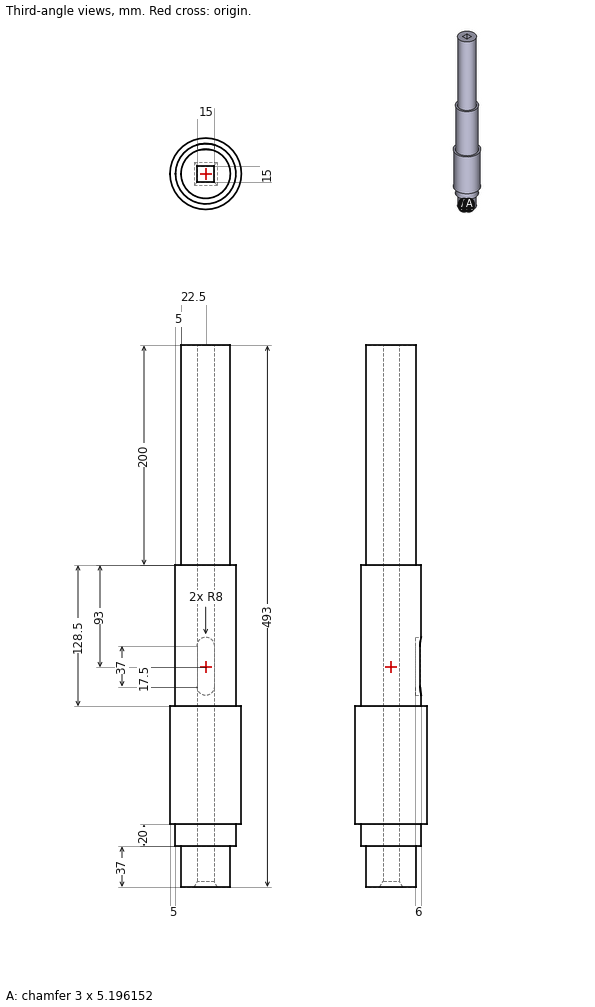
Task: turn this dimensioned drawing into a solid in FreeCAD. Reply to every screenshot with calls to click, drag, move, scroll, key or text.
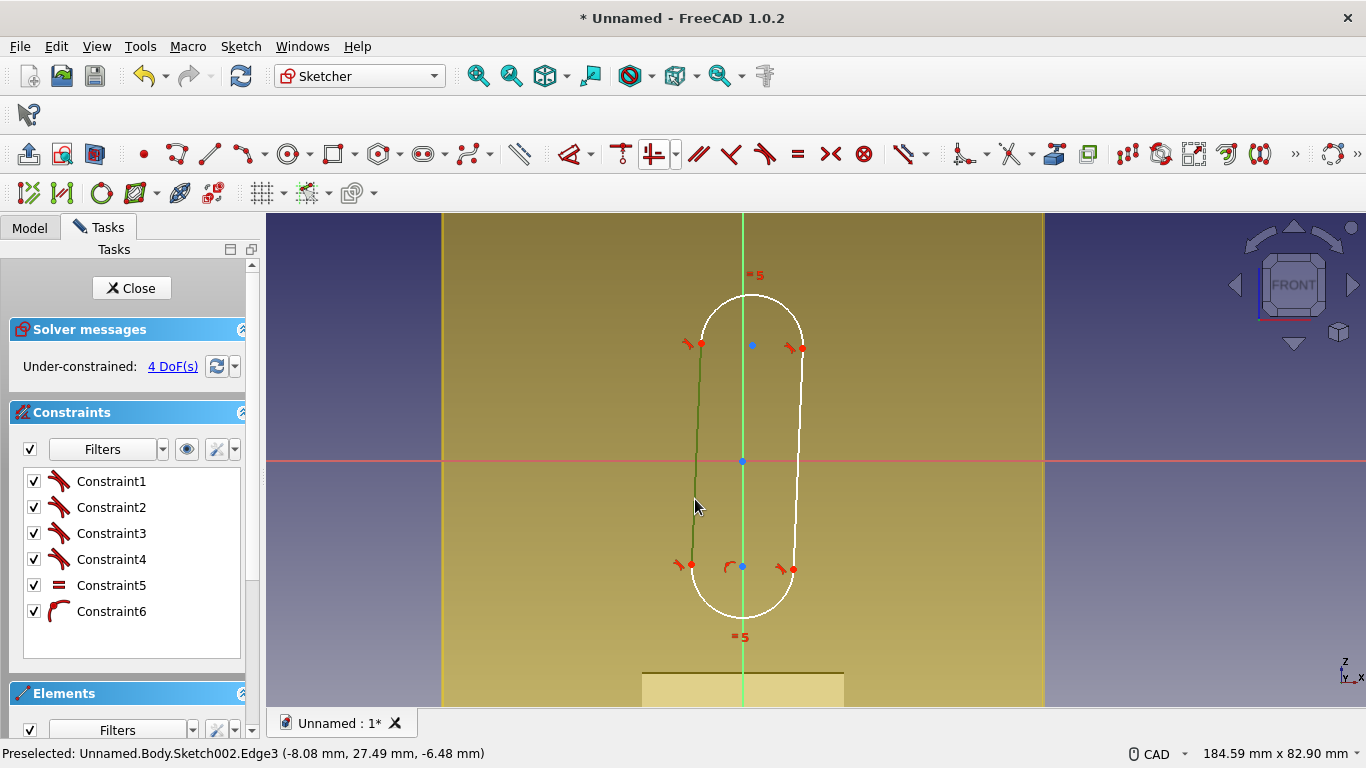
key(v)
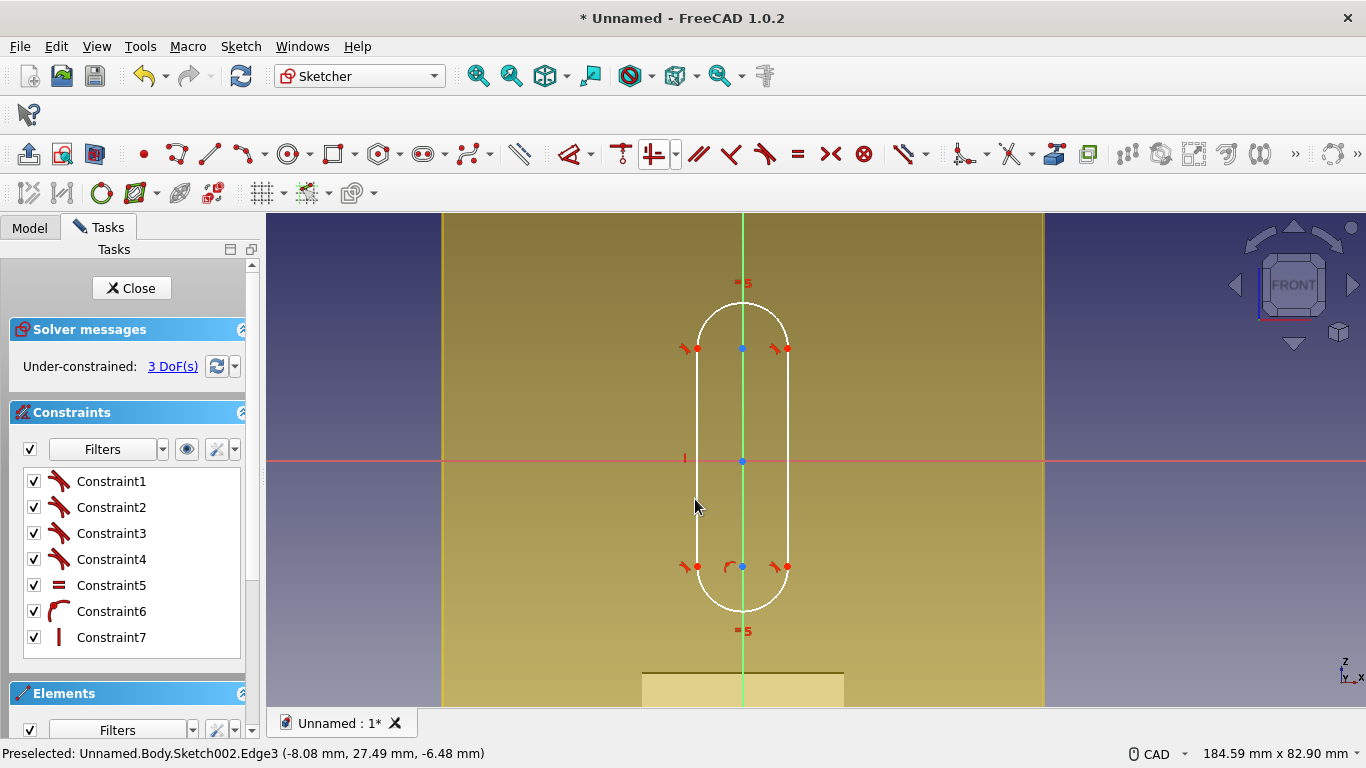
key(d)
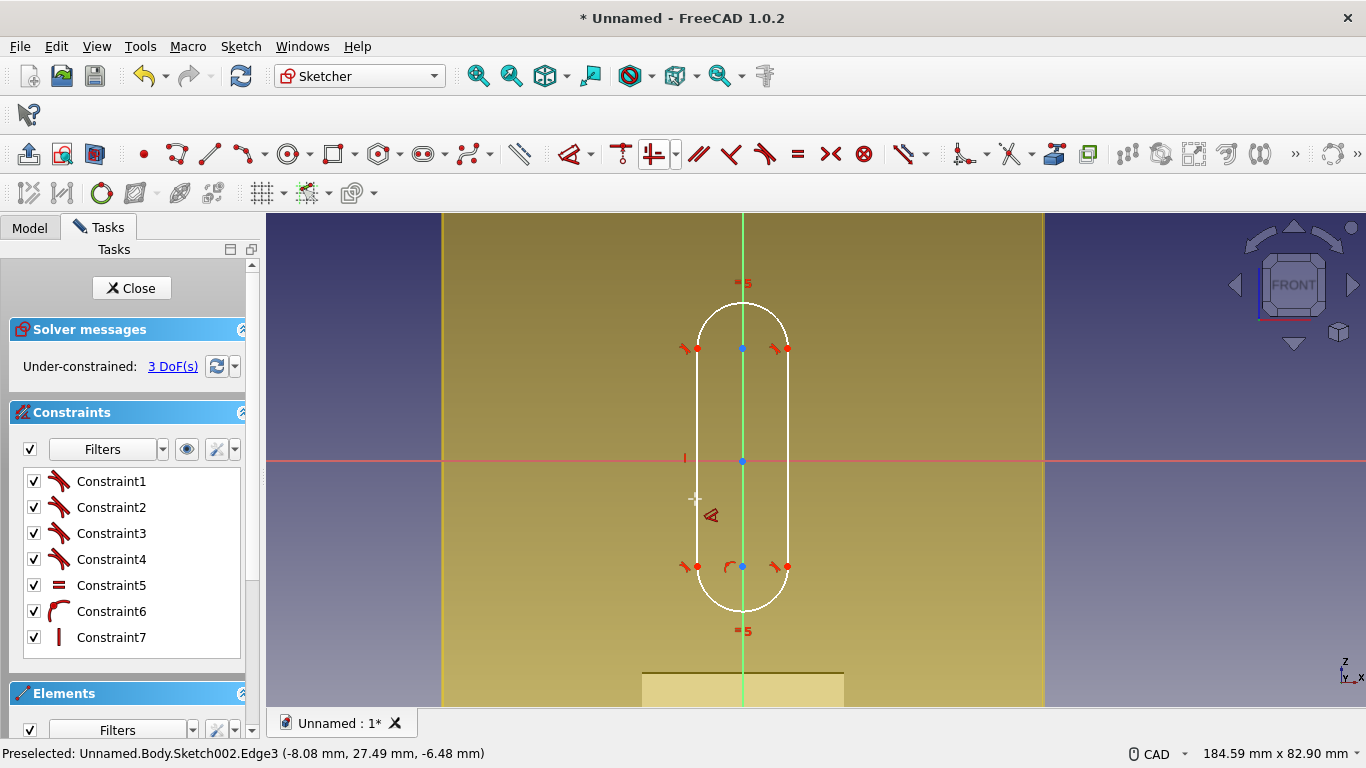
click(716, 603)
click(697, 629)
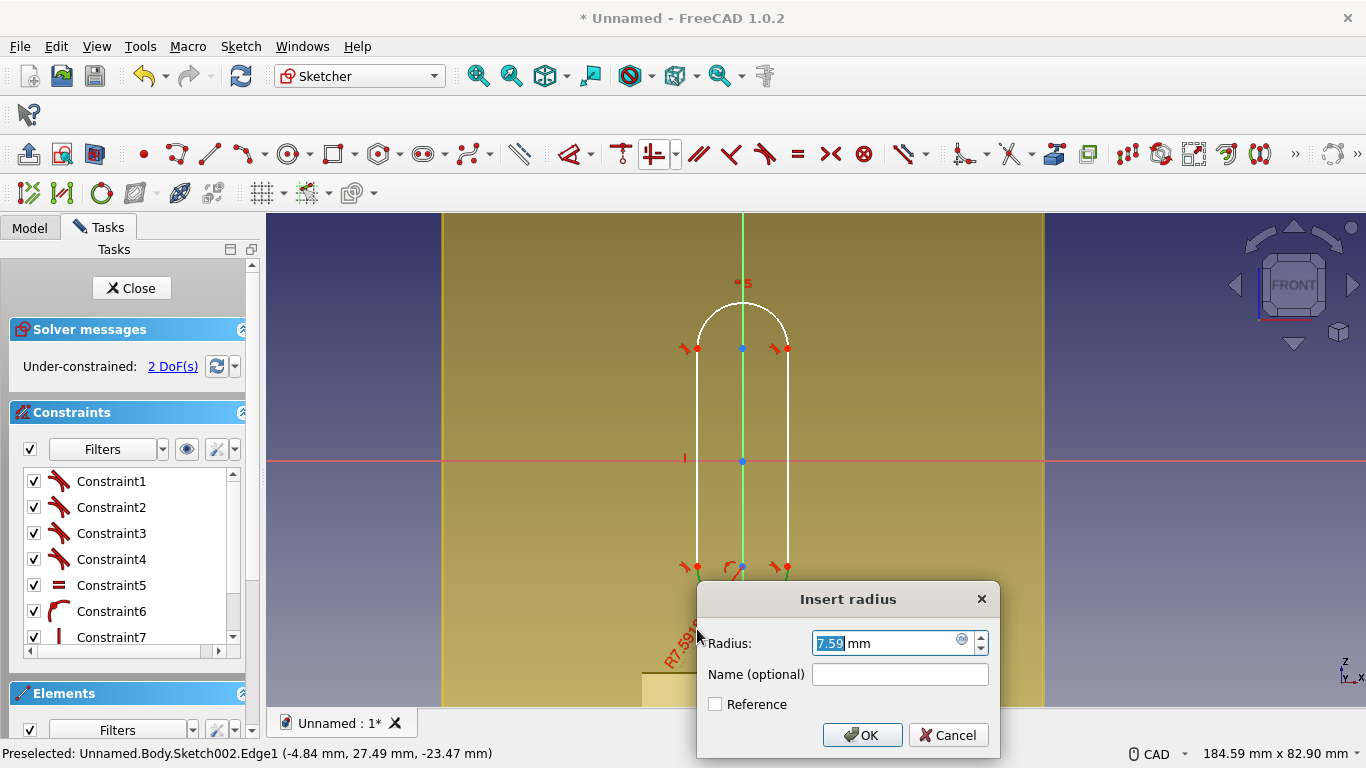
text(8)
key(Return)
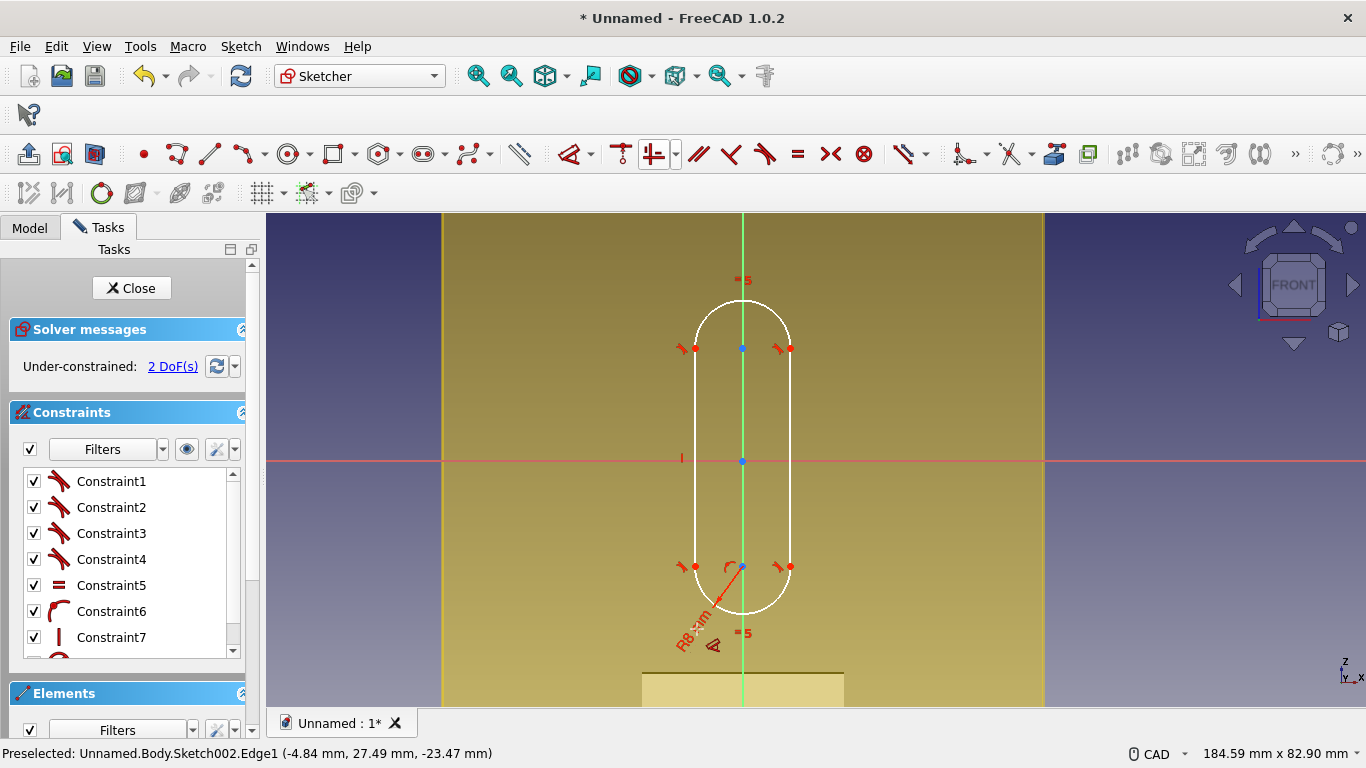
click(695, 501)
click(661, 407)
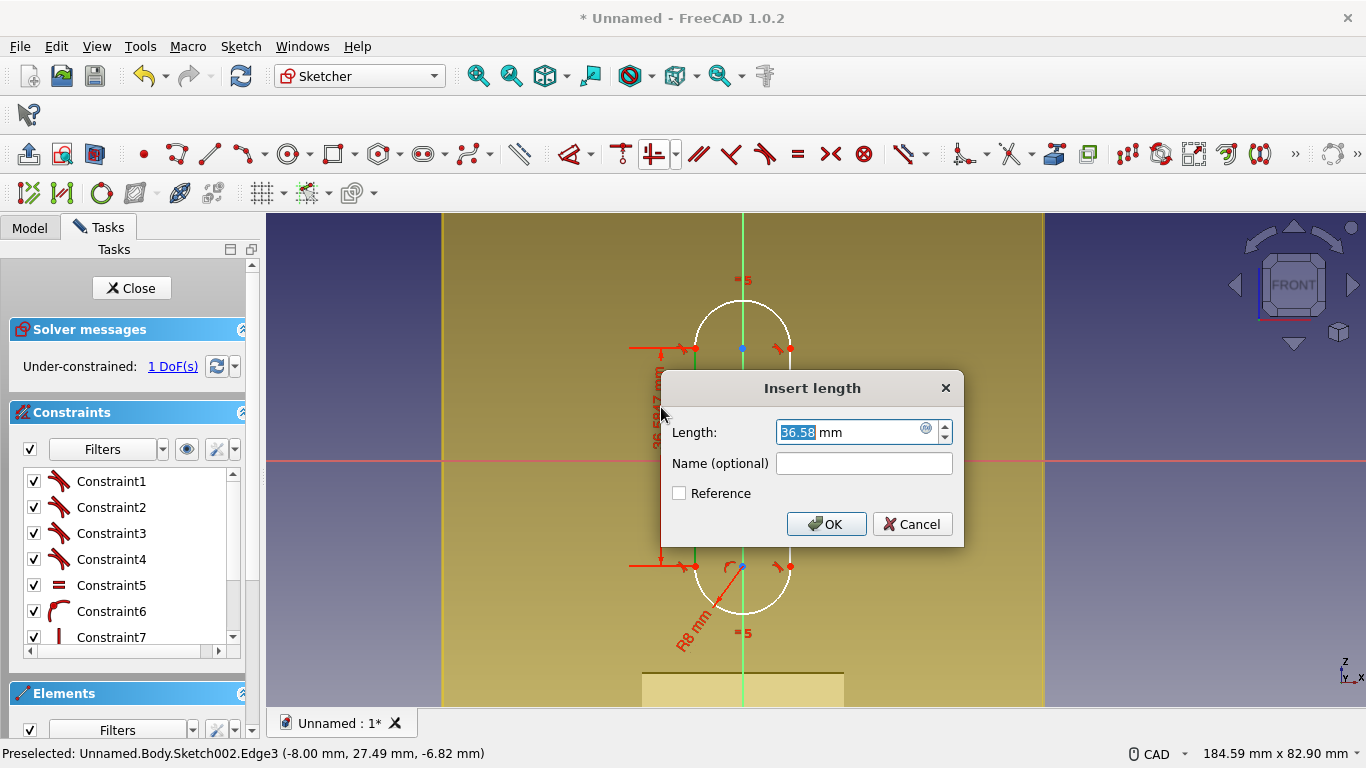
text(37)
key(Return)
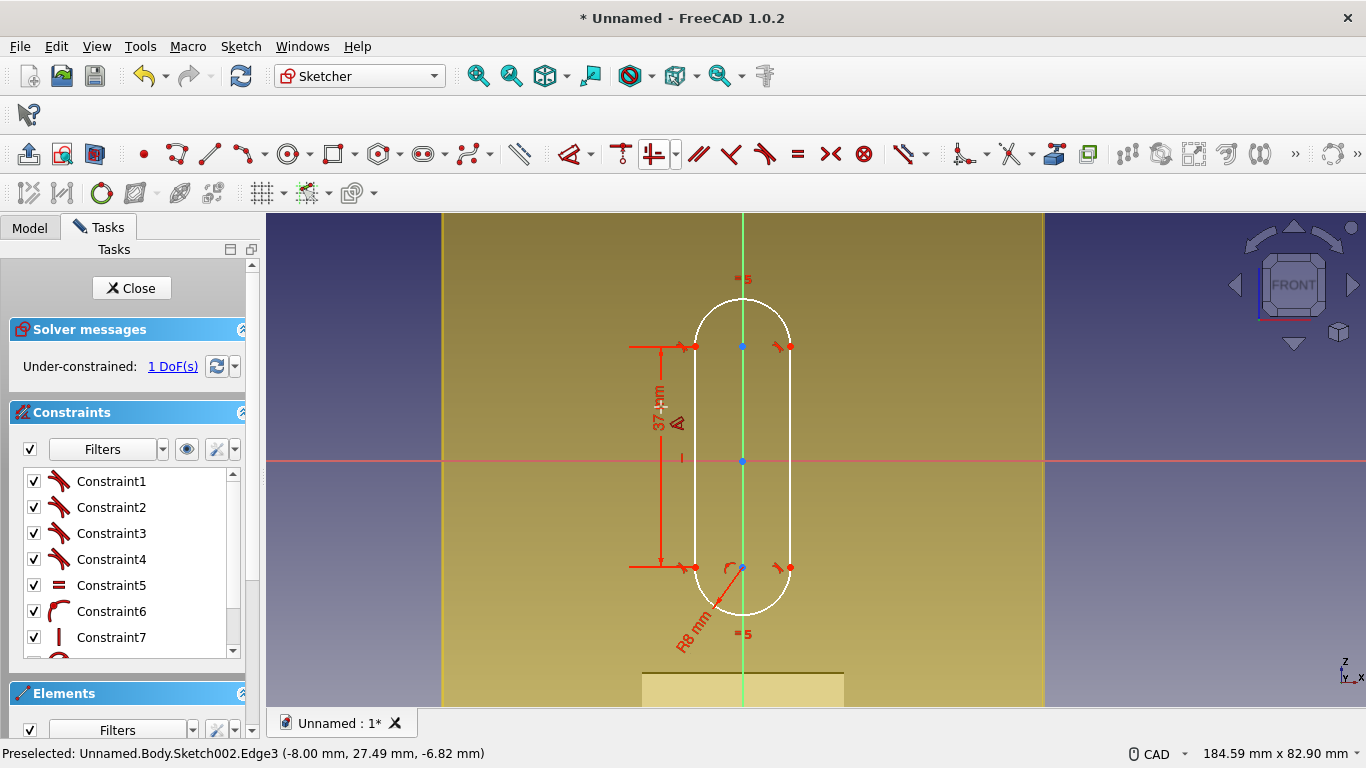
click(695, 567)
click(661, 514)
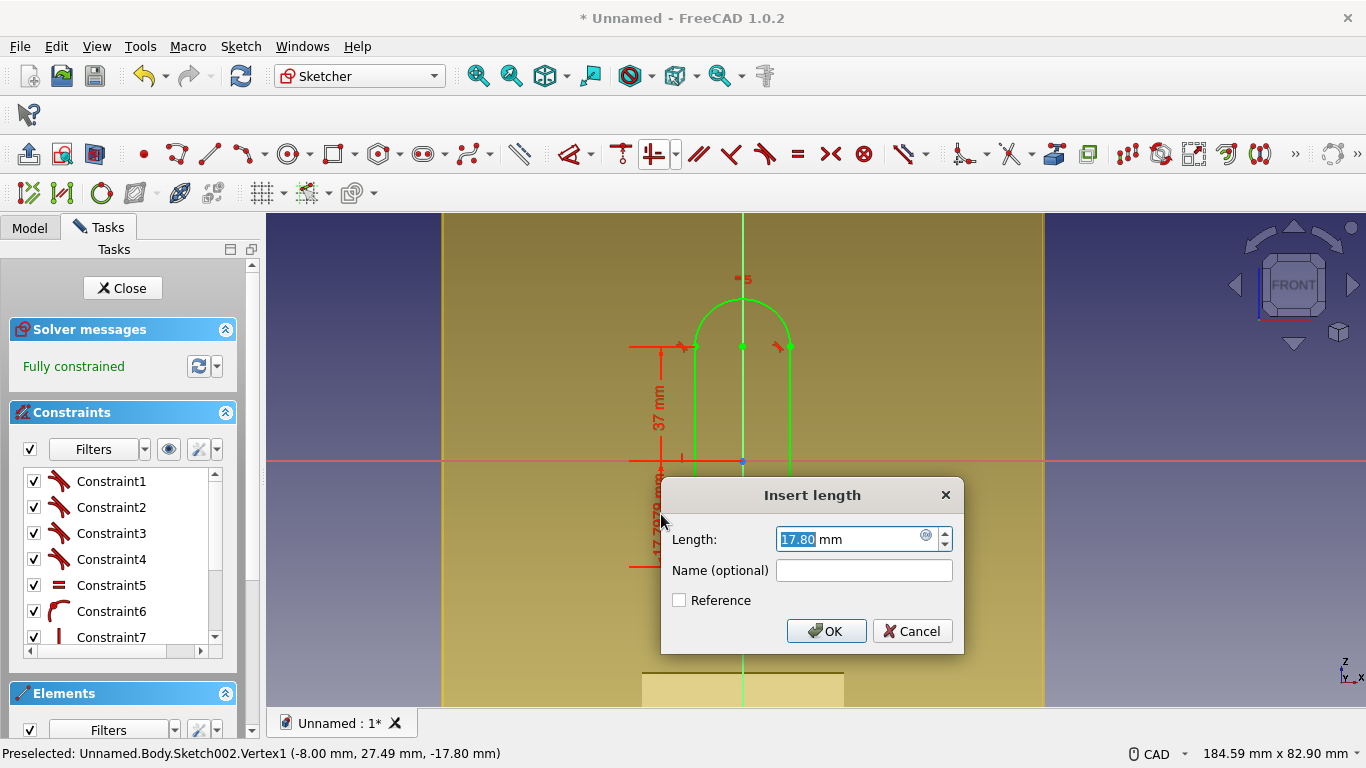
text(17.5)
key(Return)
key(Escape)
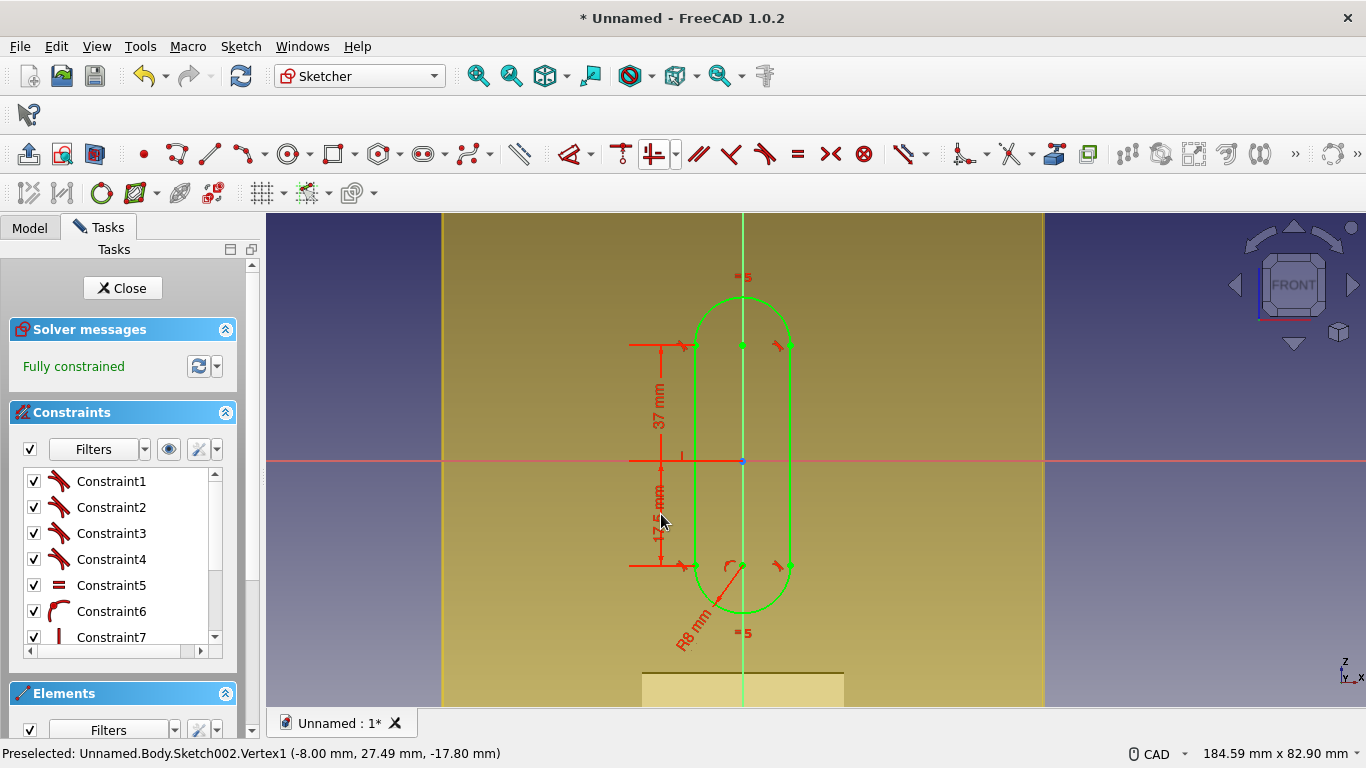
click(123, 288)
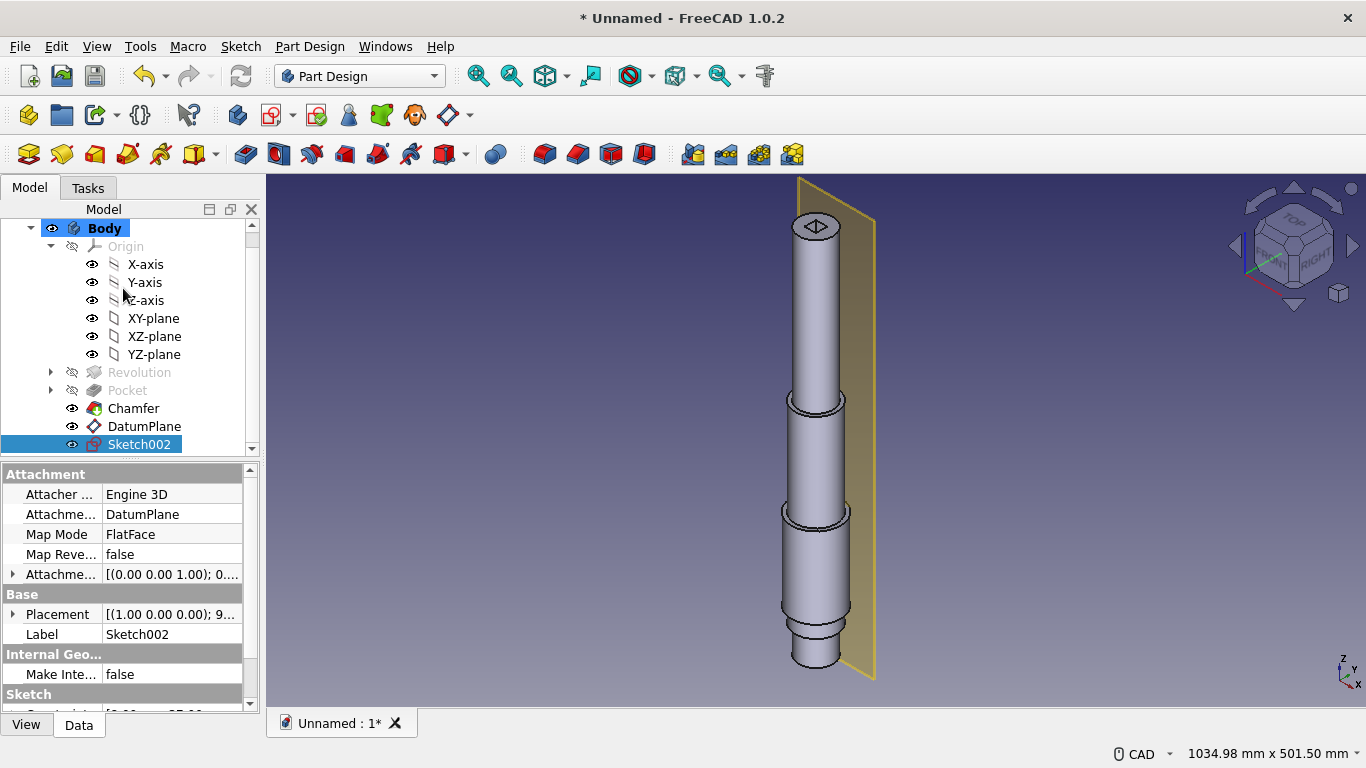
click(246, 154)